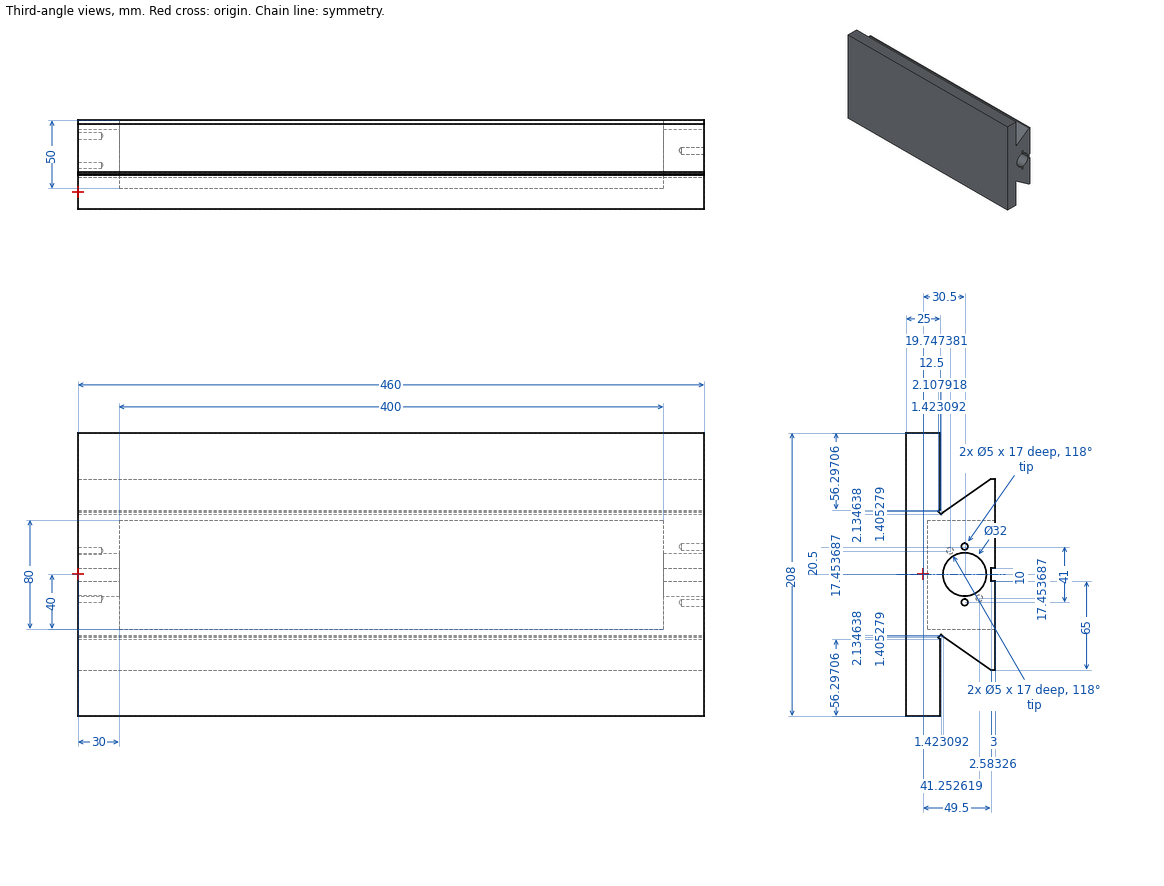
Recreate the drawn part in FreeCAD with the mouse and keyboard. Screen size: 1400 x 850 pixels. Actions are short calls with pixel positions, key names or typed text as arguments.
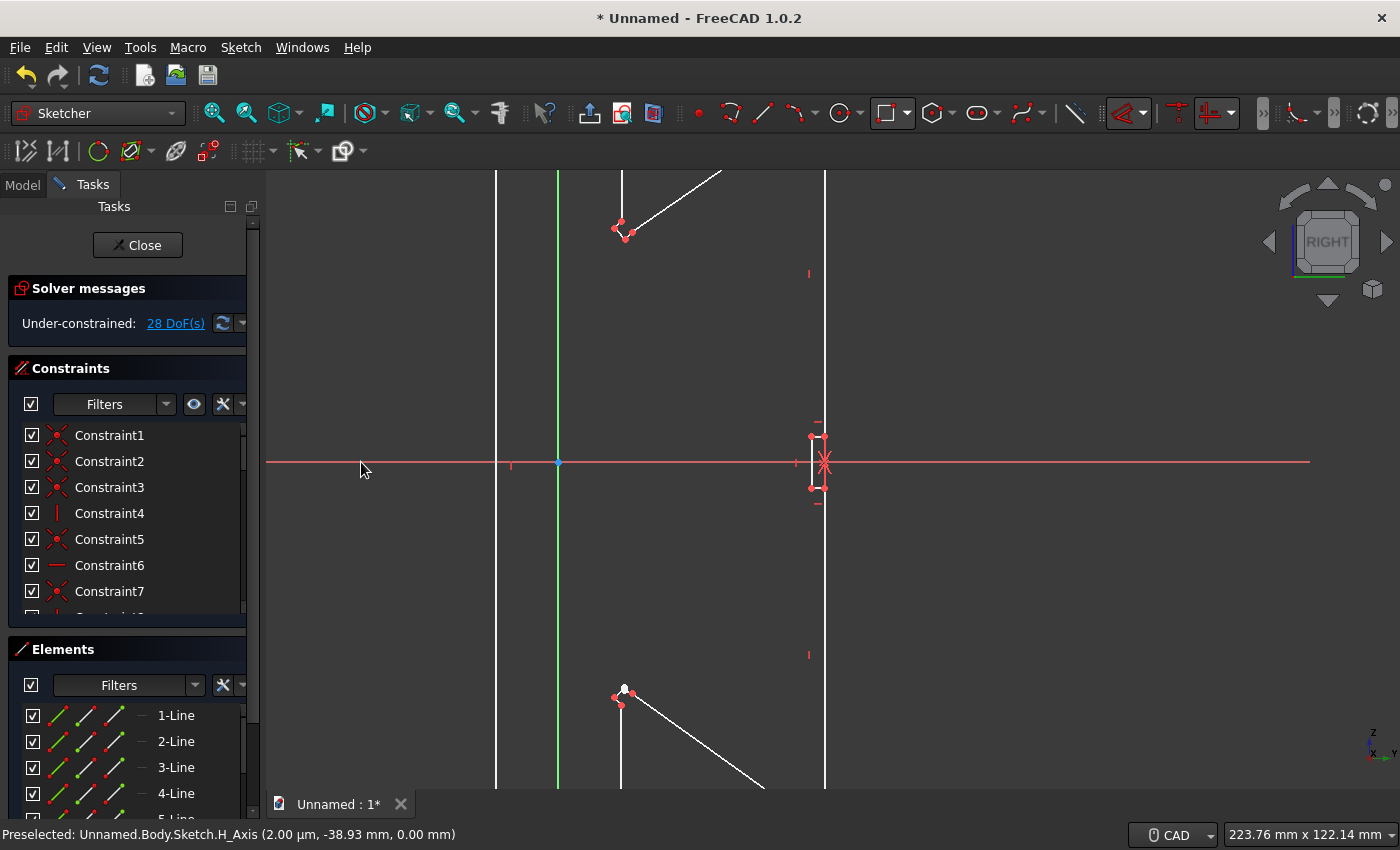
scroll(826, 489, down, 5)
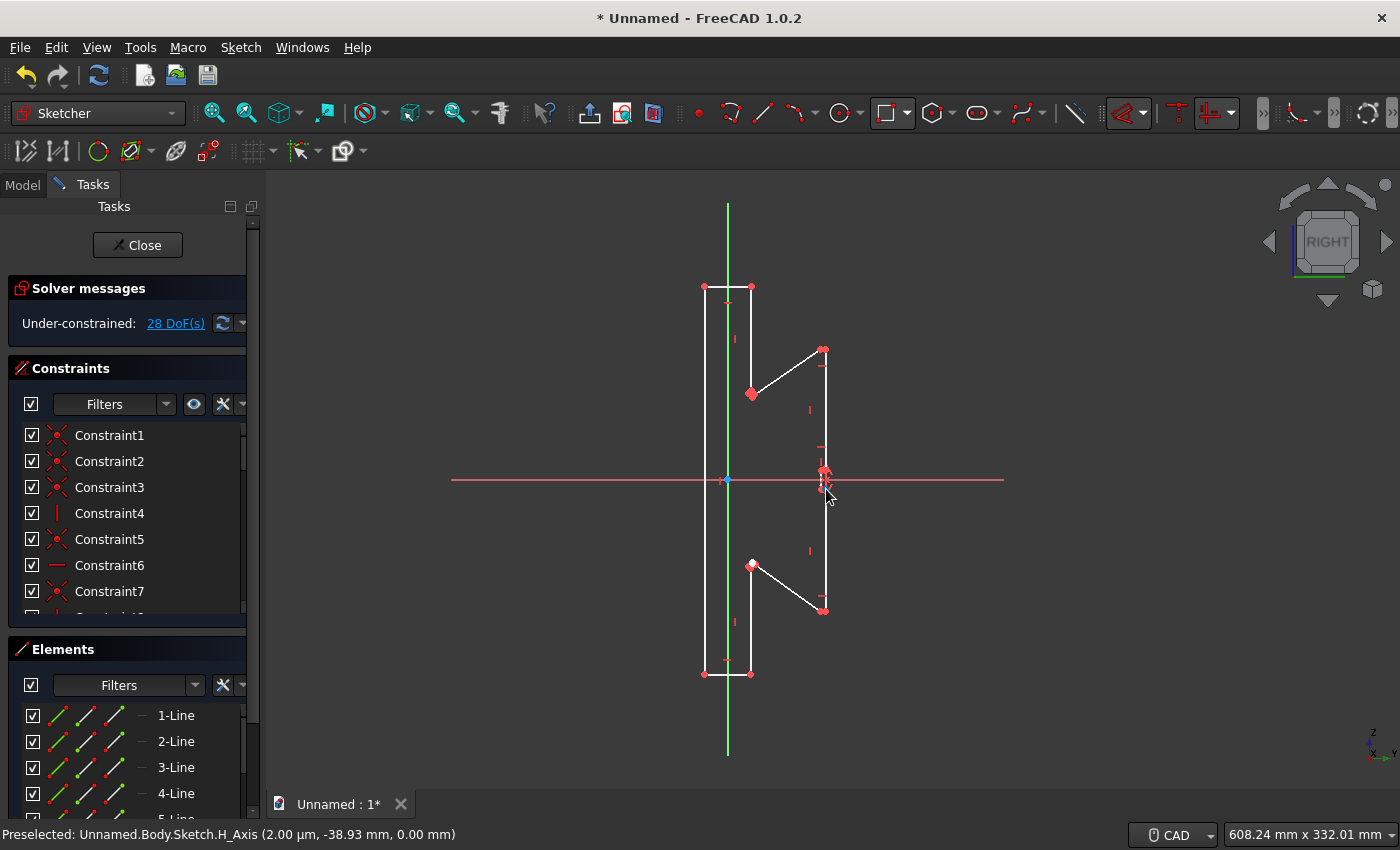
scroll(820, 611, up, 4)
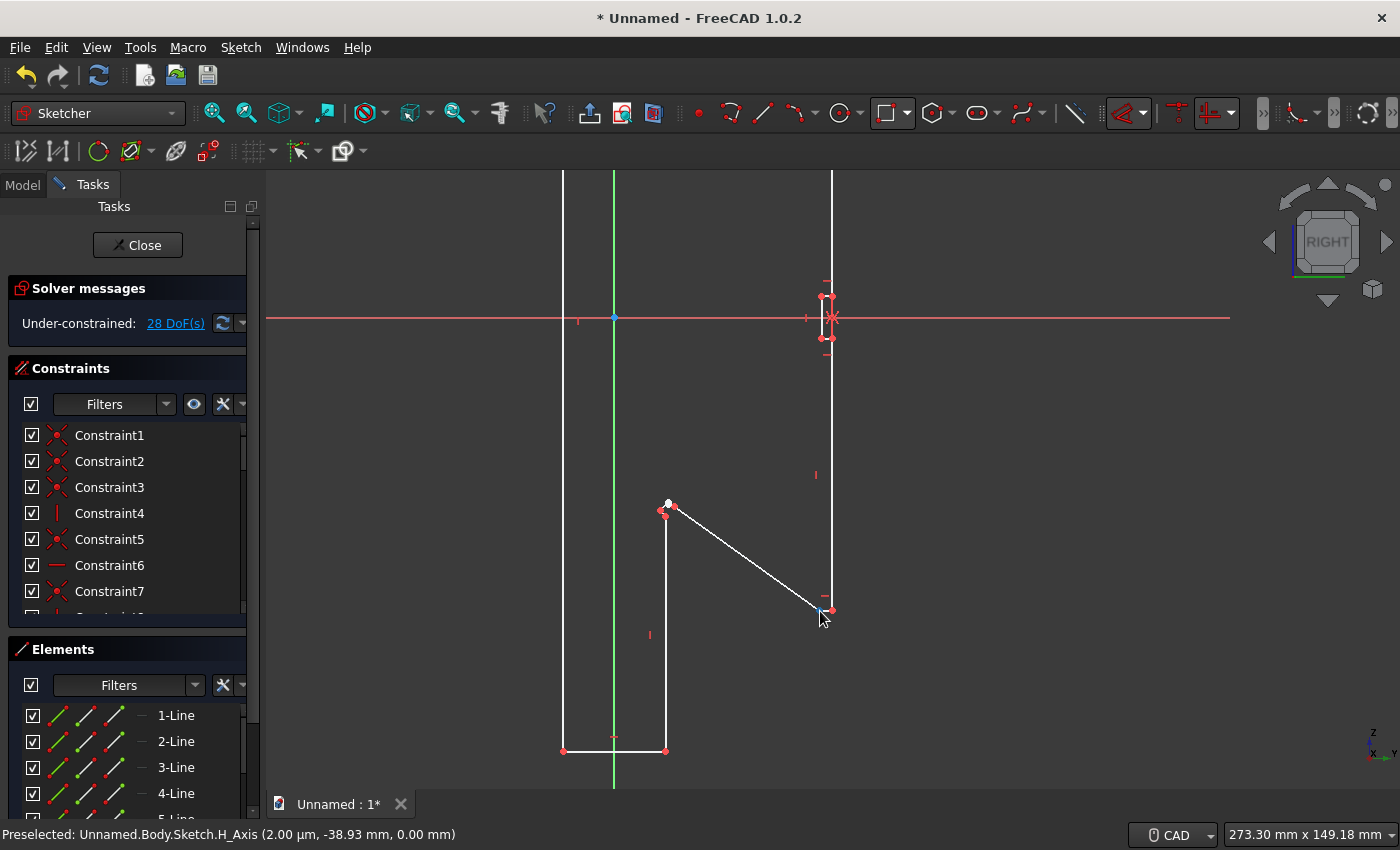
click(820, 611)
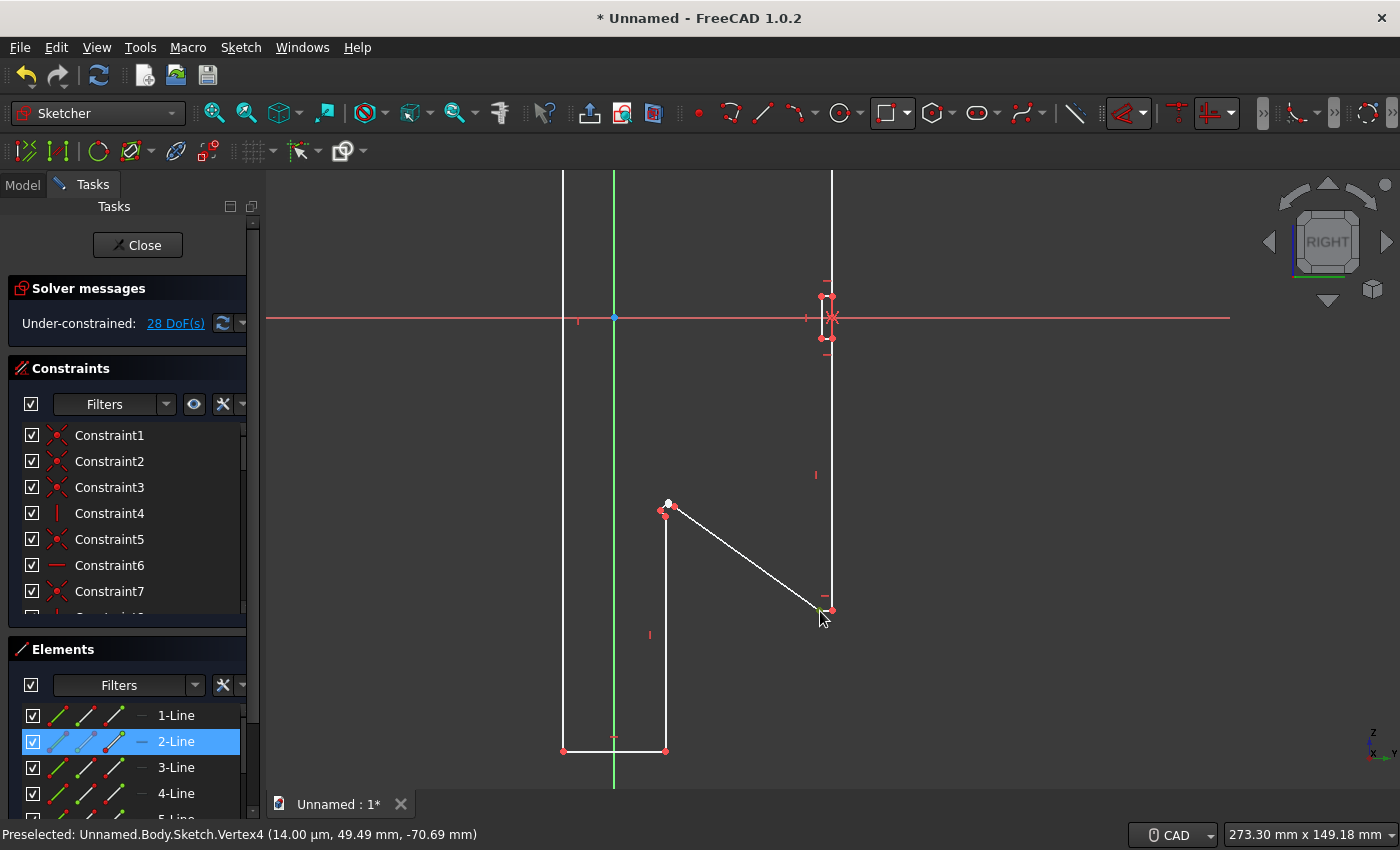
scroll(819, 612, down, 4)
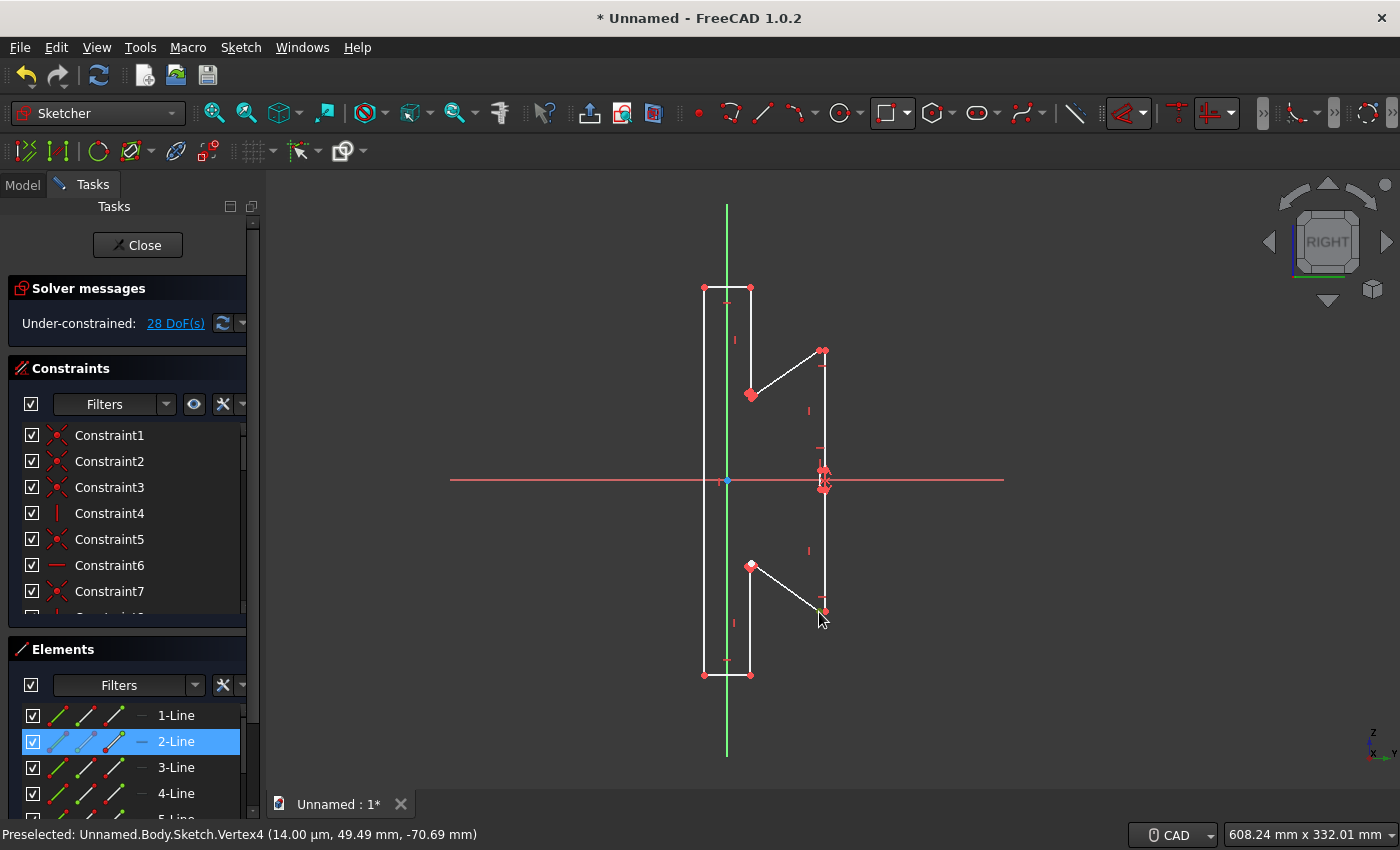
scroll(819, 350, up, 4)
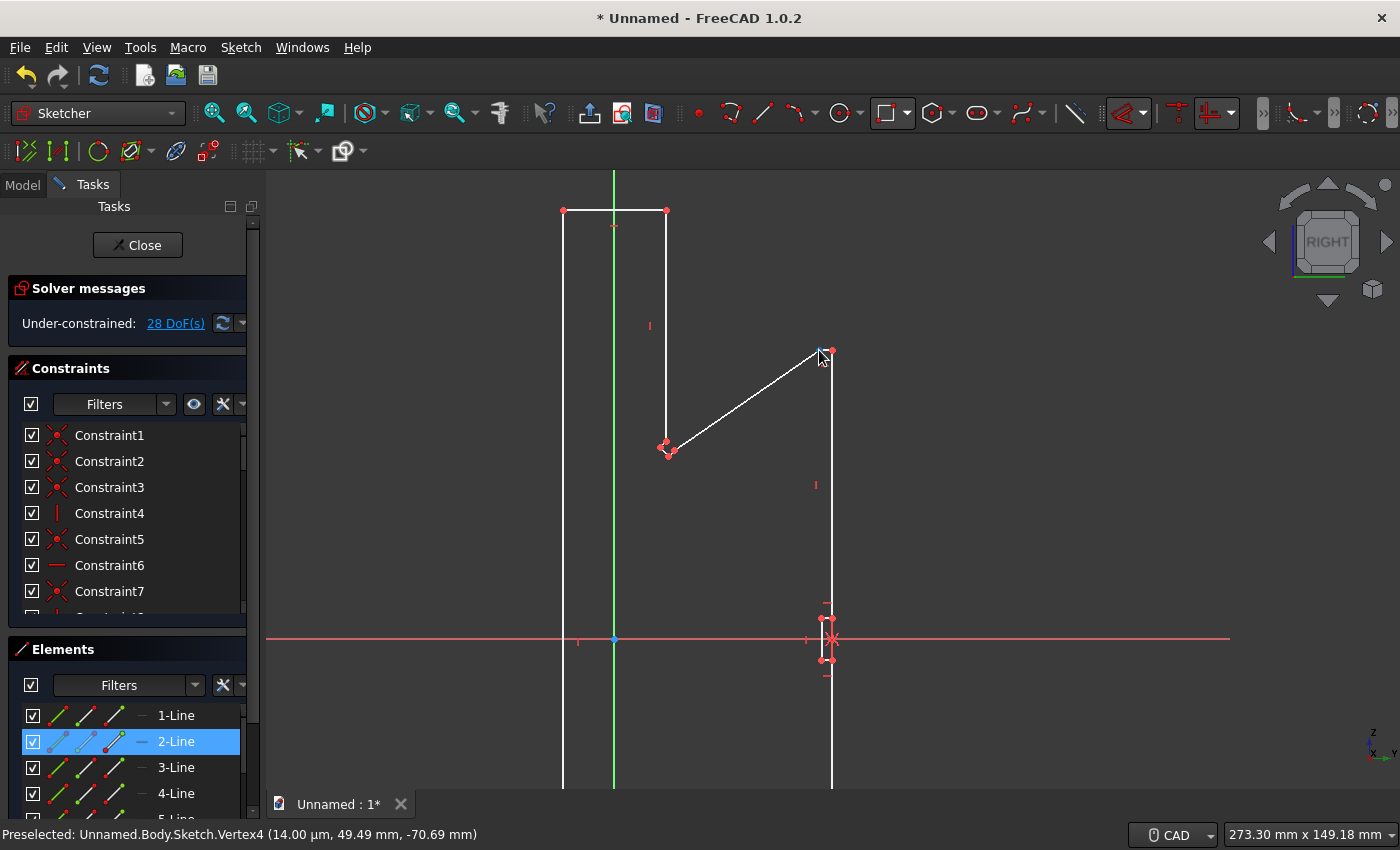
click(819, 350)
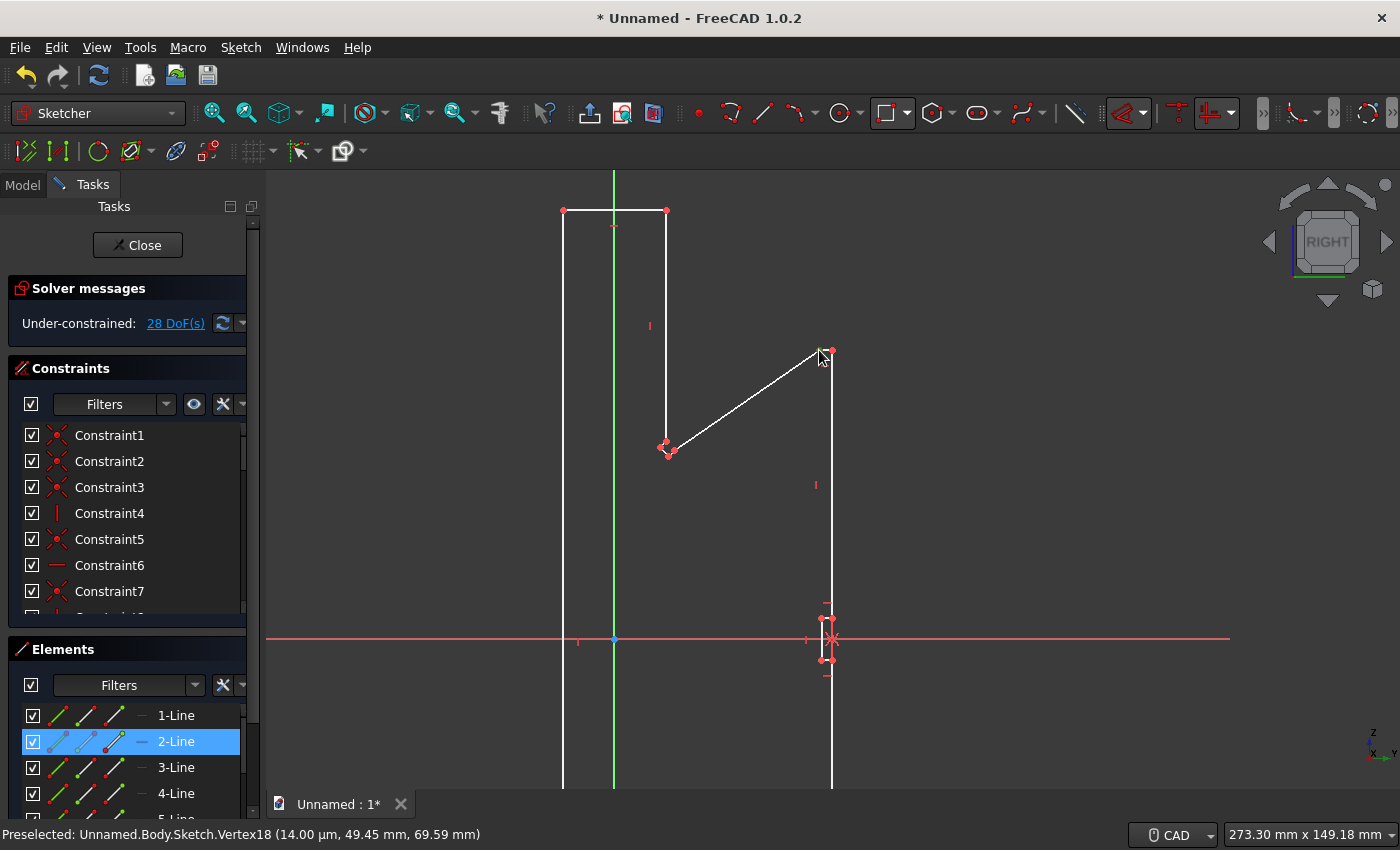
click(361, 639)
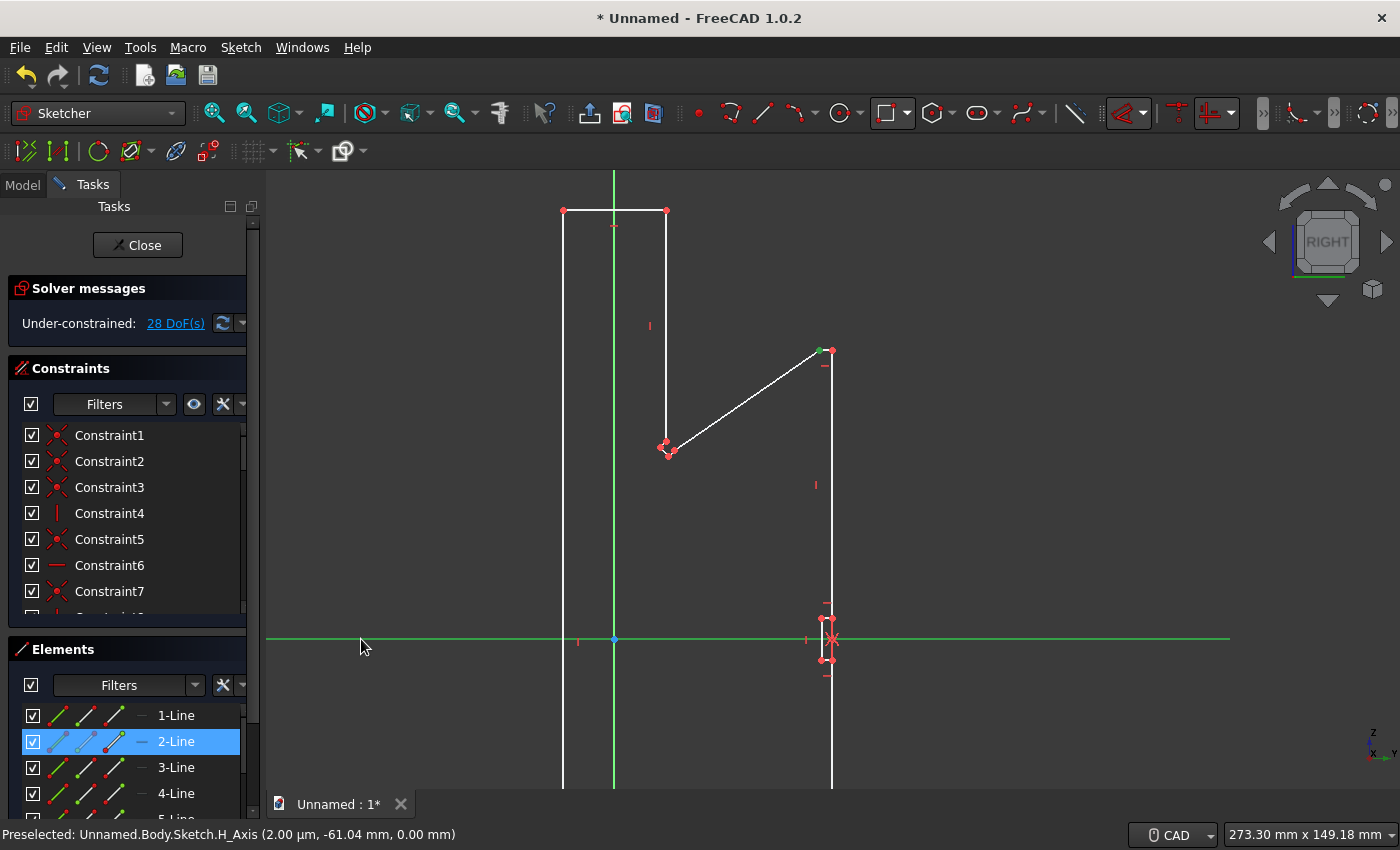
key(s)